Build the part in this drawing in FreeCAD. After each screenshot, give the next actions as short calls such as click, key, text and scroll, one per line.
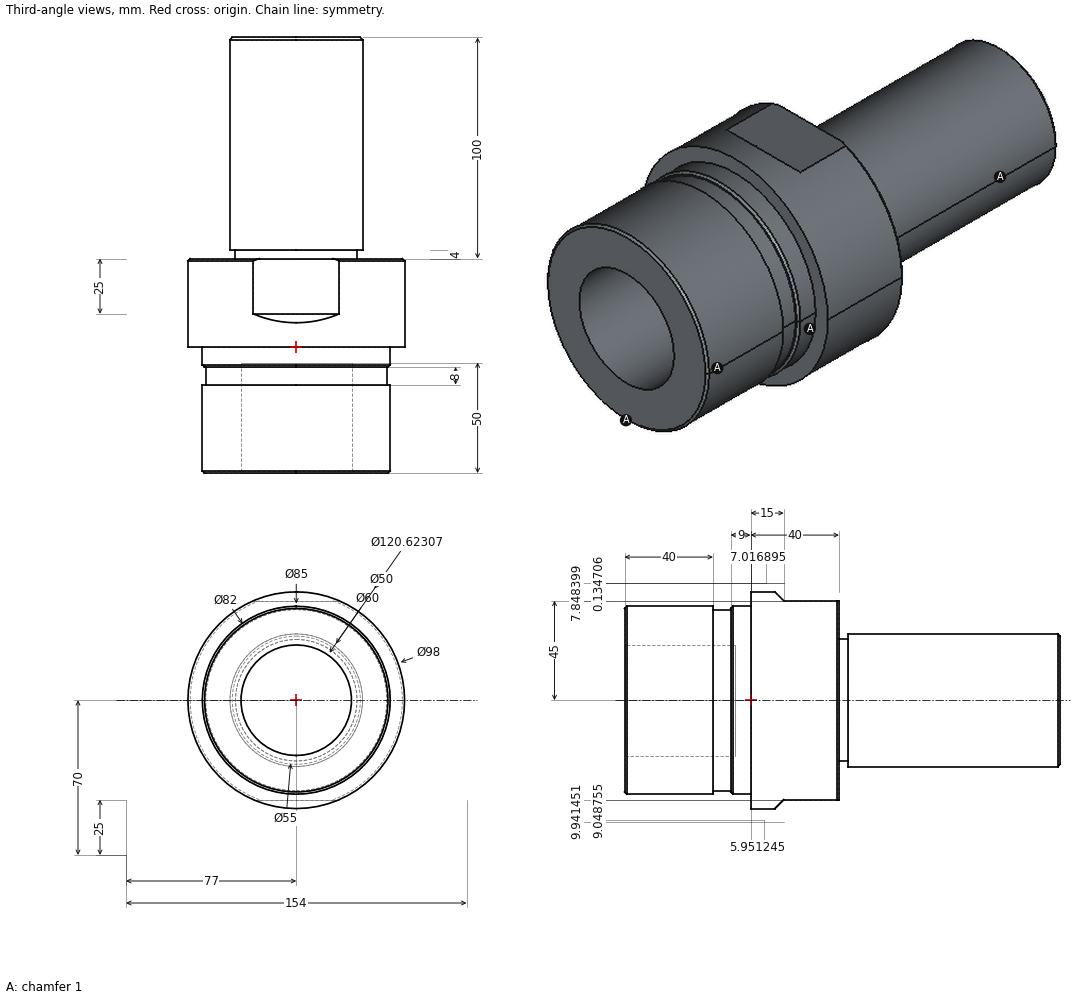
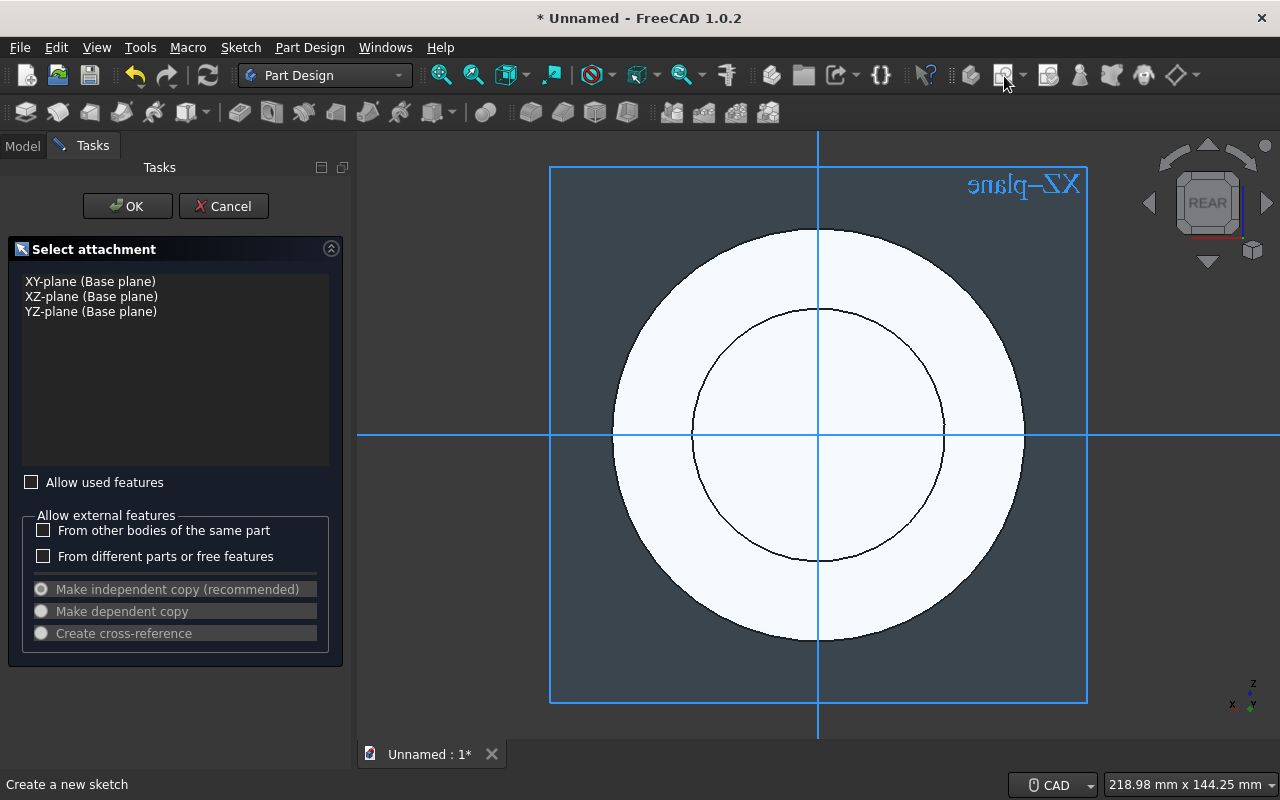
click(82, 296)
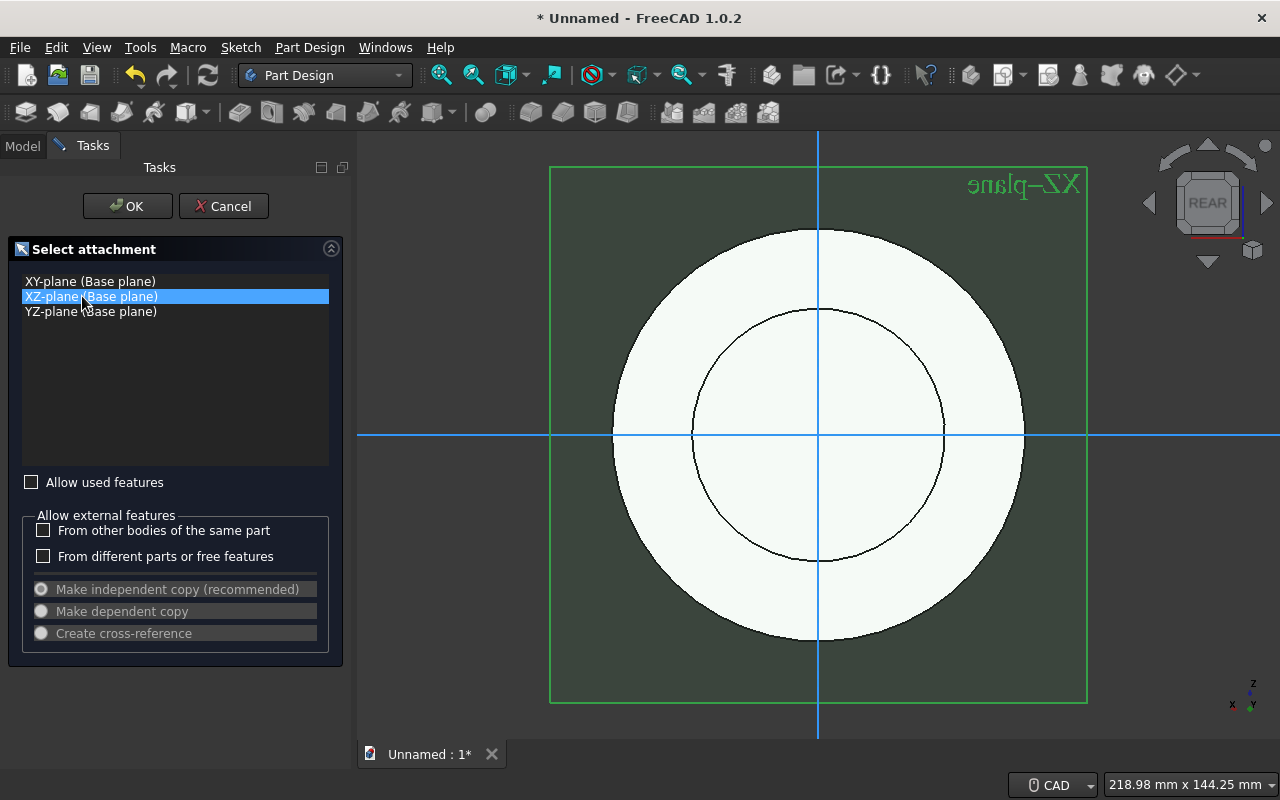
click(128, 206)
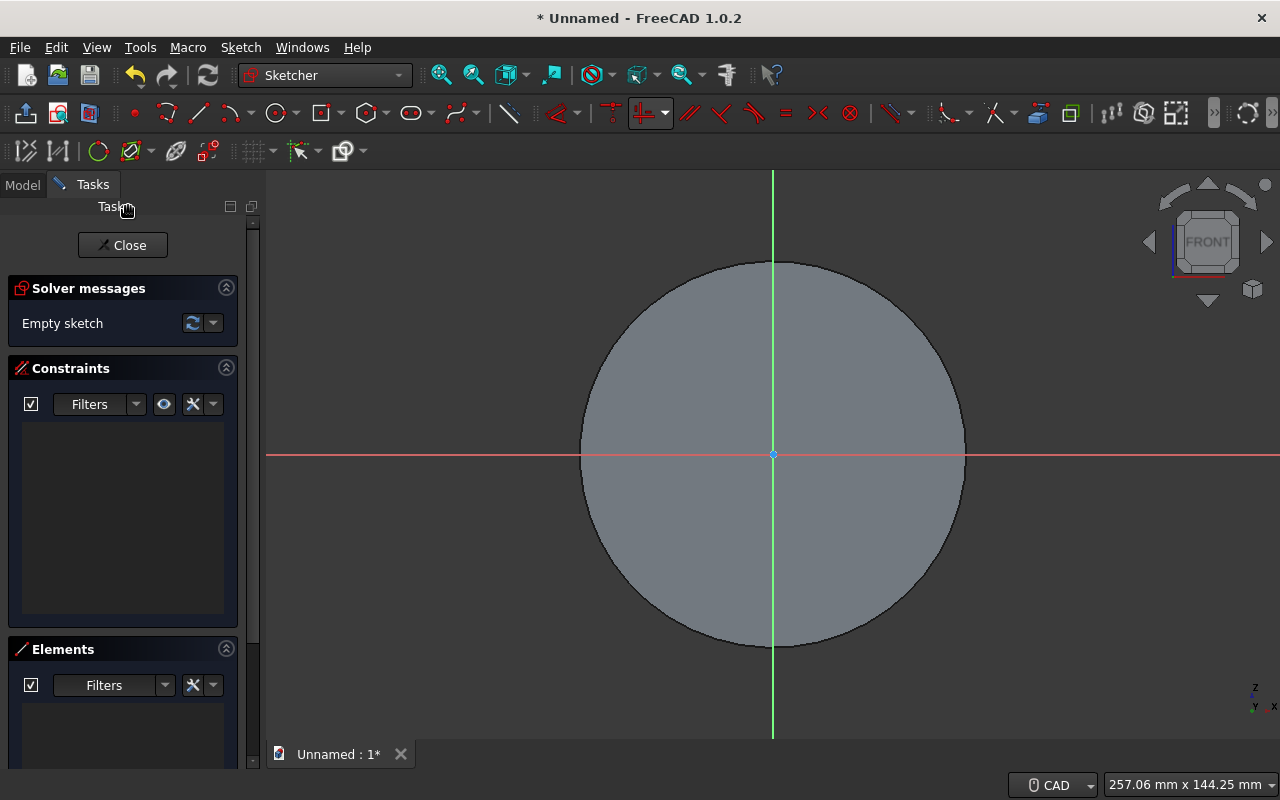
click(276, 114)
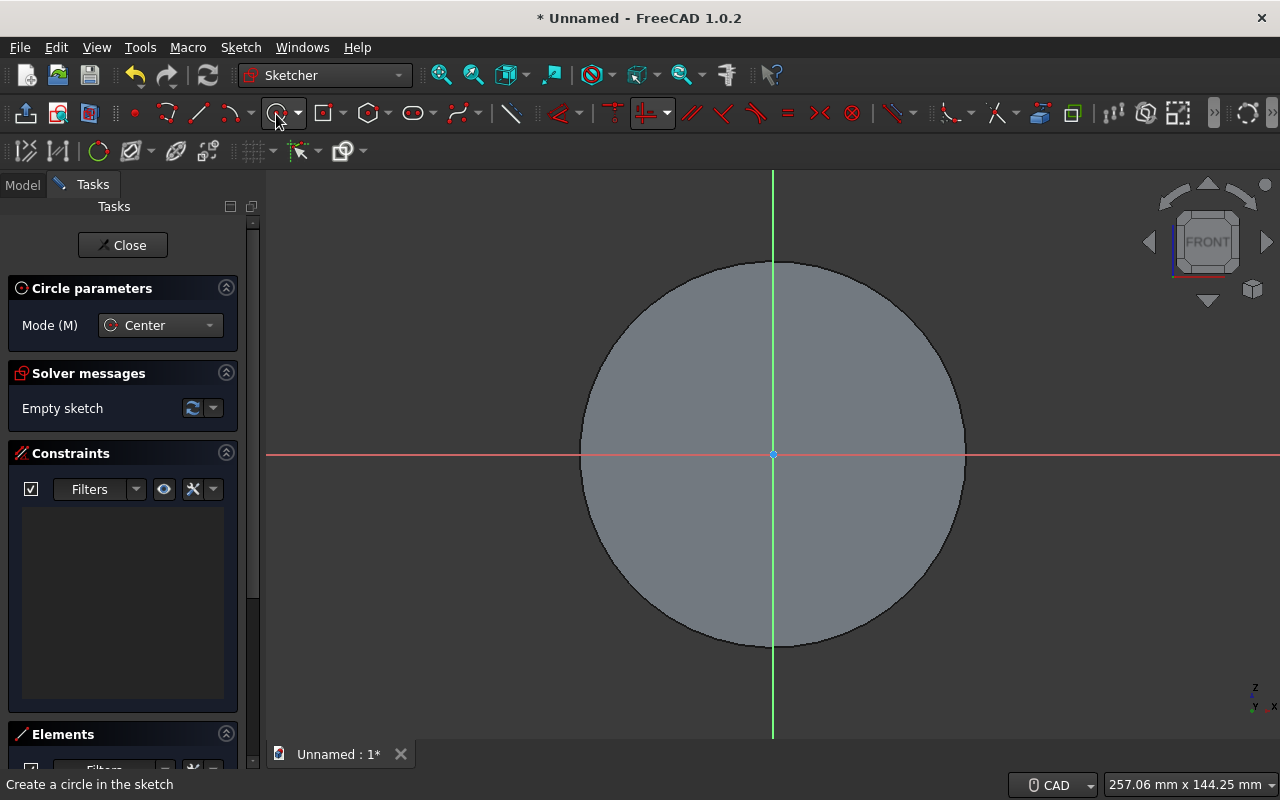
click(773, 455)
click(892, 336)
key(Escape)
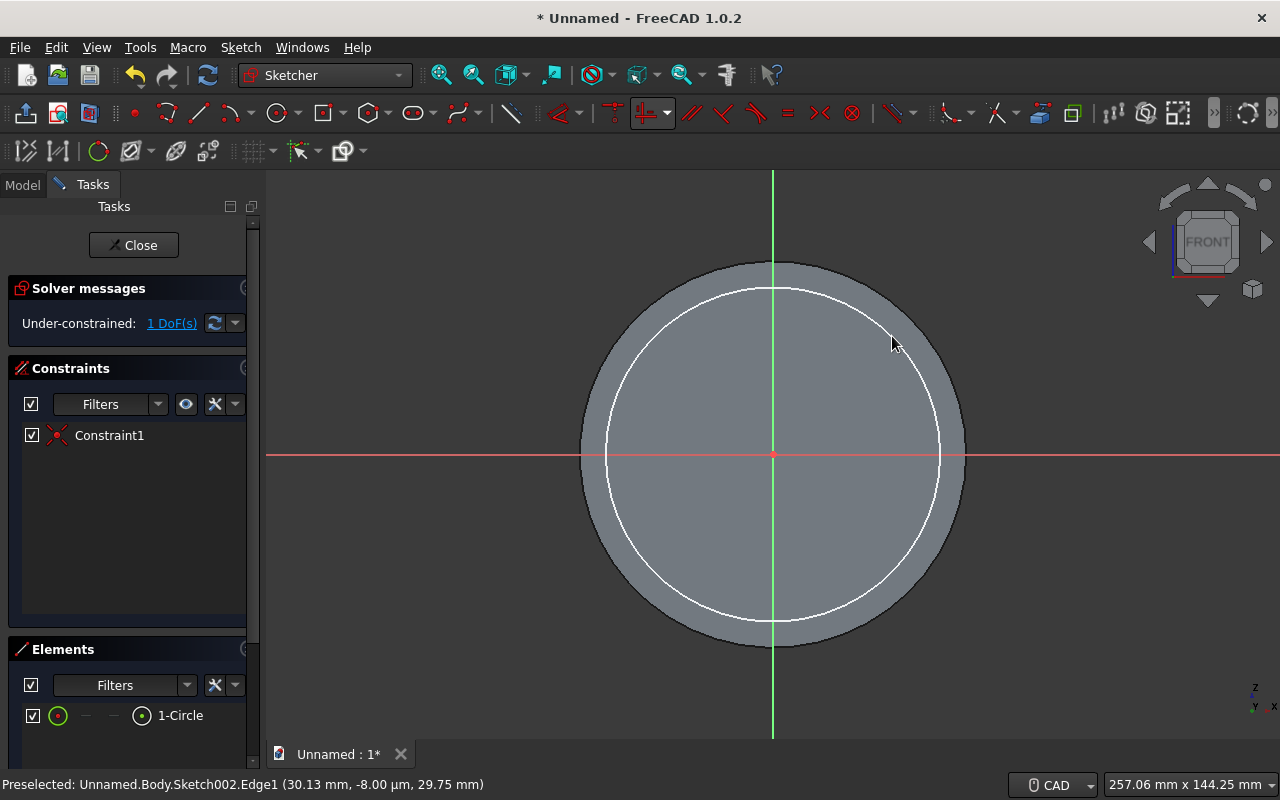
click(558, 114)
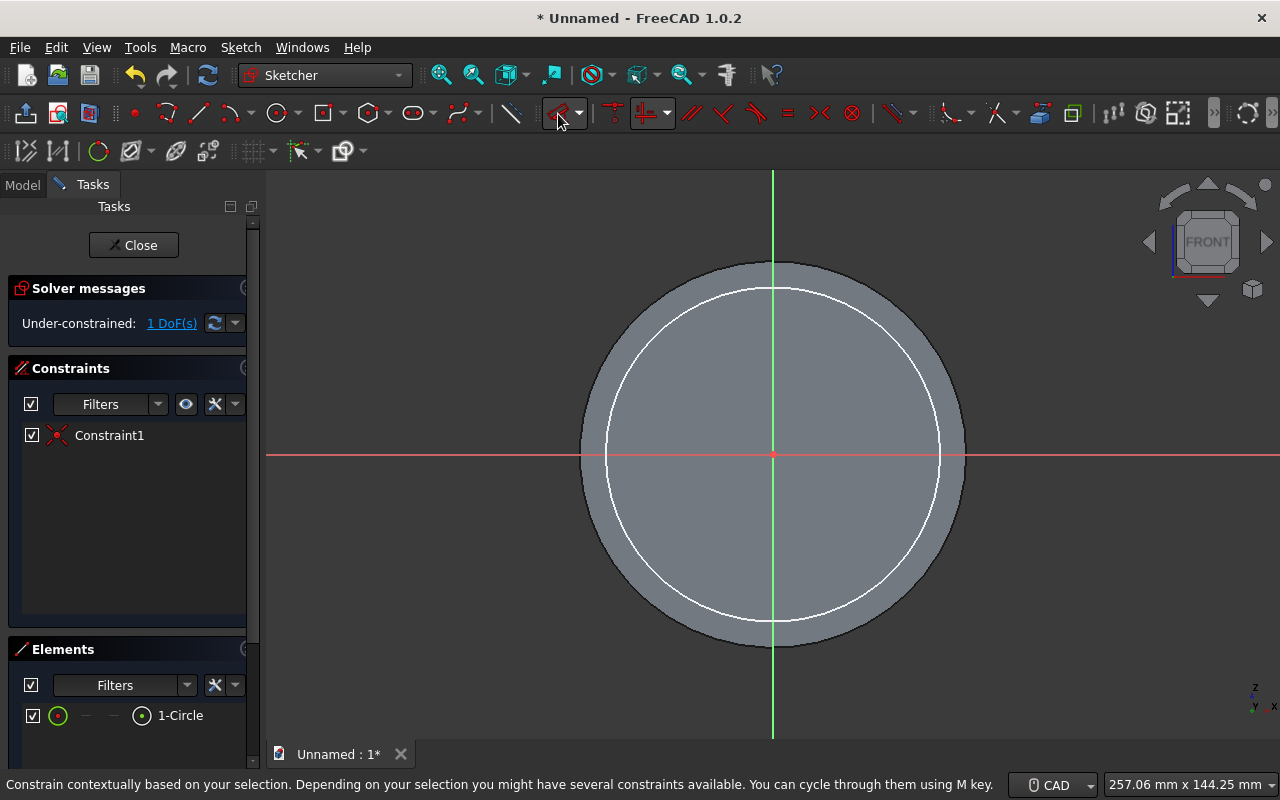
click(891, 336)
click(914, 313)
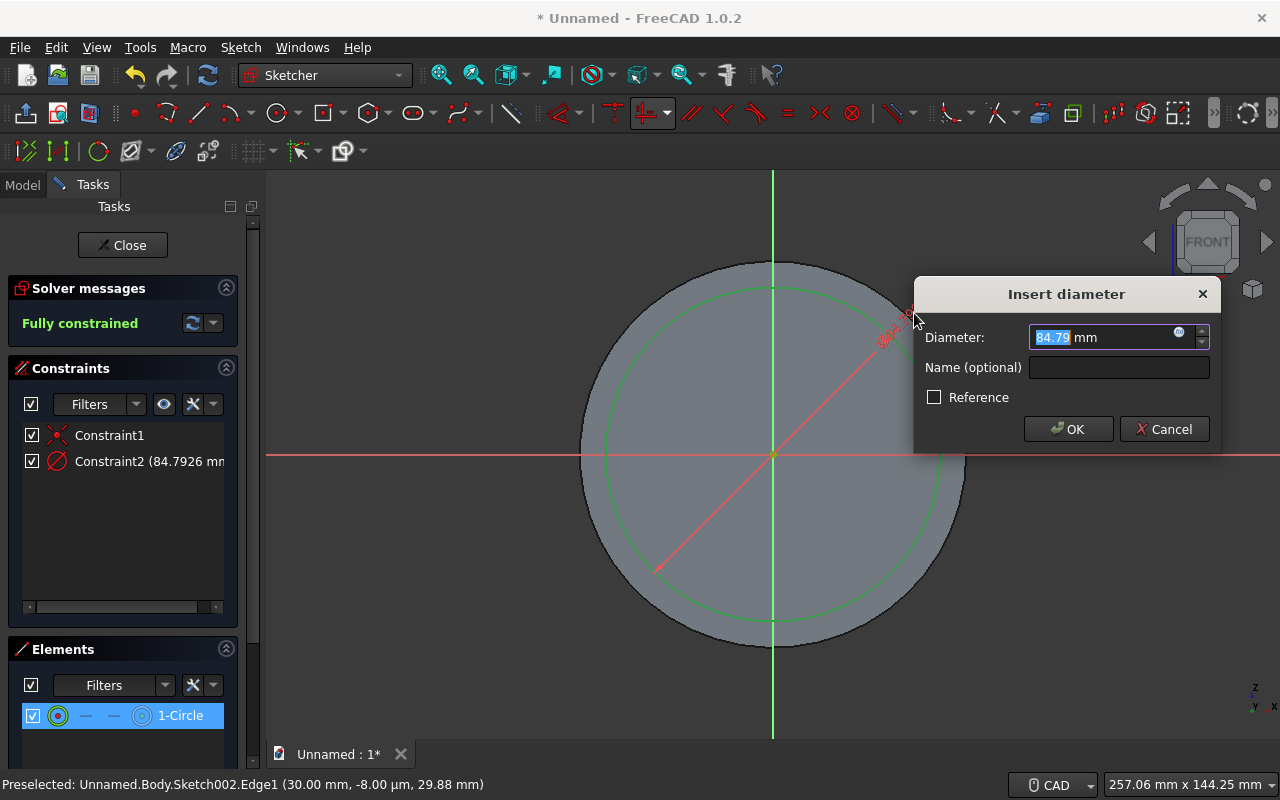
text(85)
key(Return)
key(Escape)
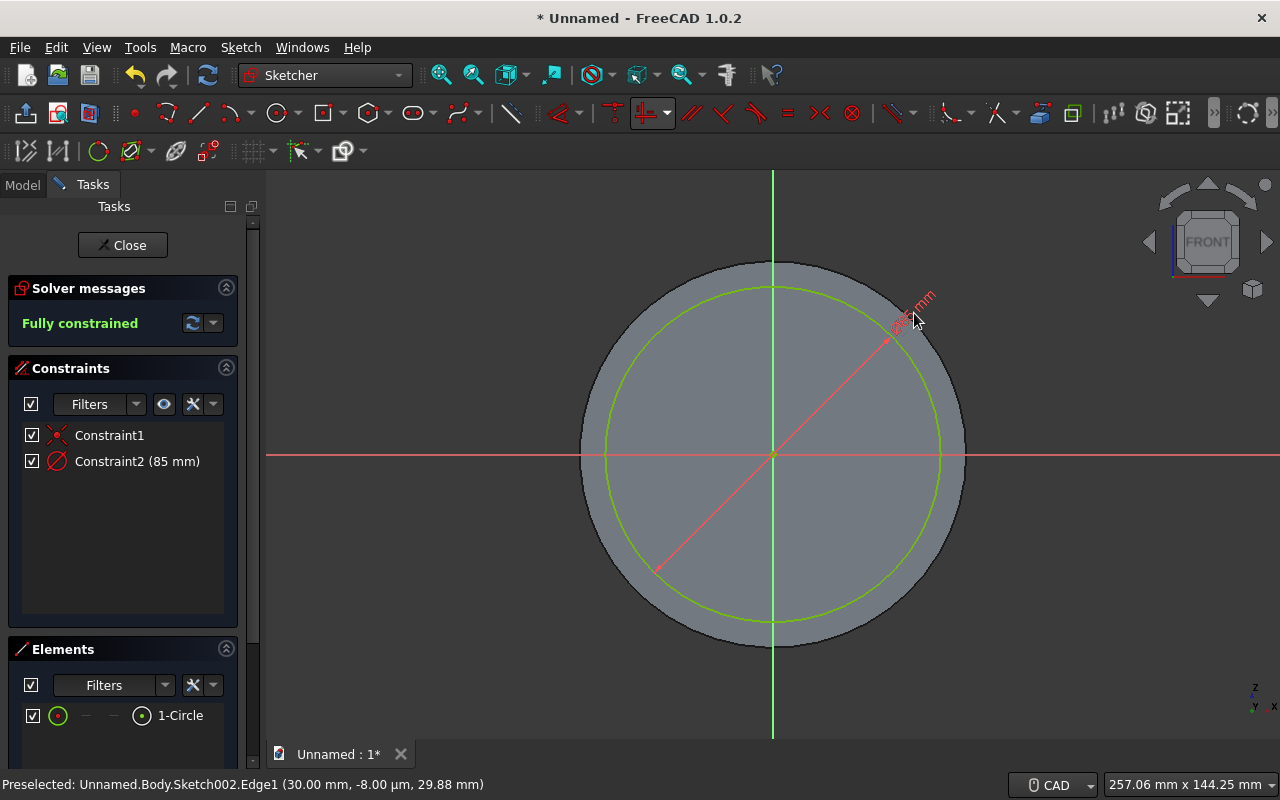
click(123, 245)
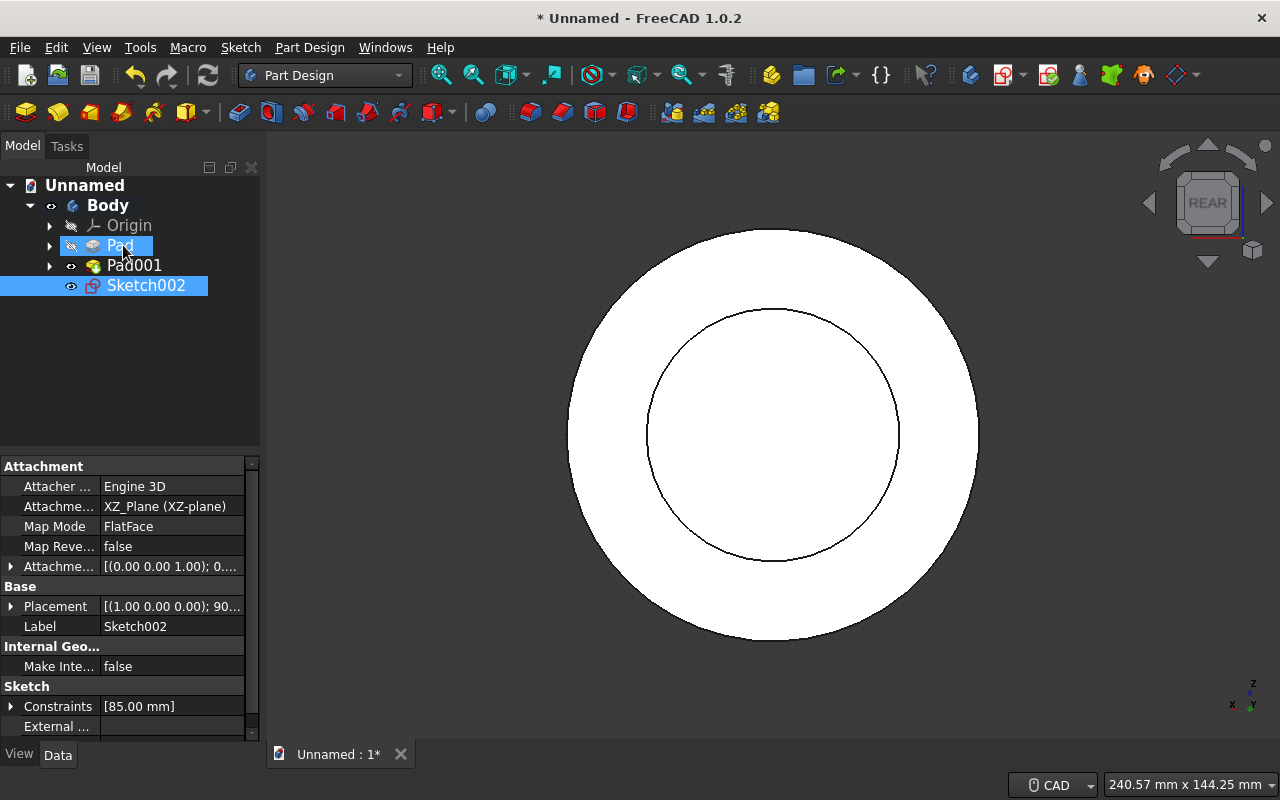
click(26, 112)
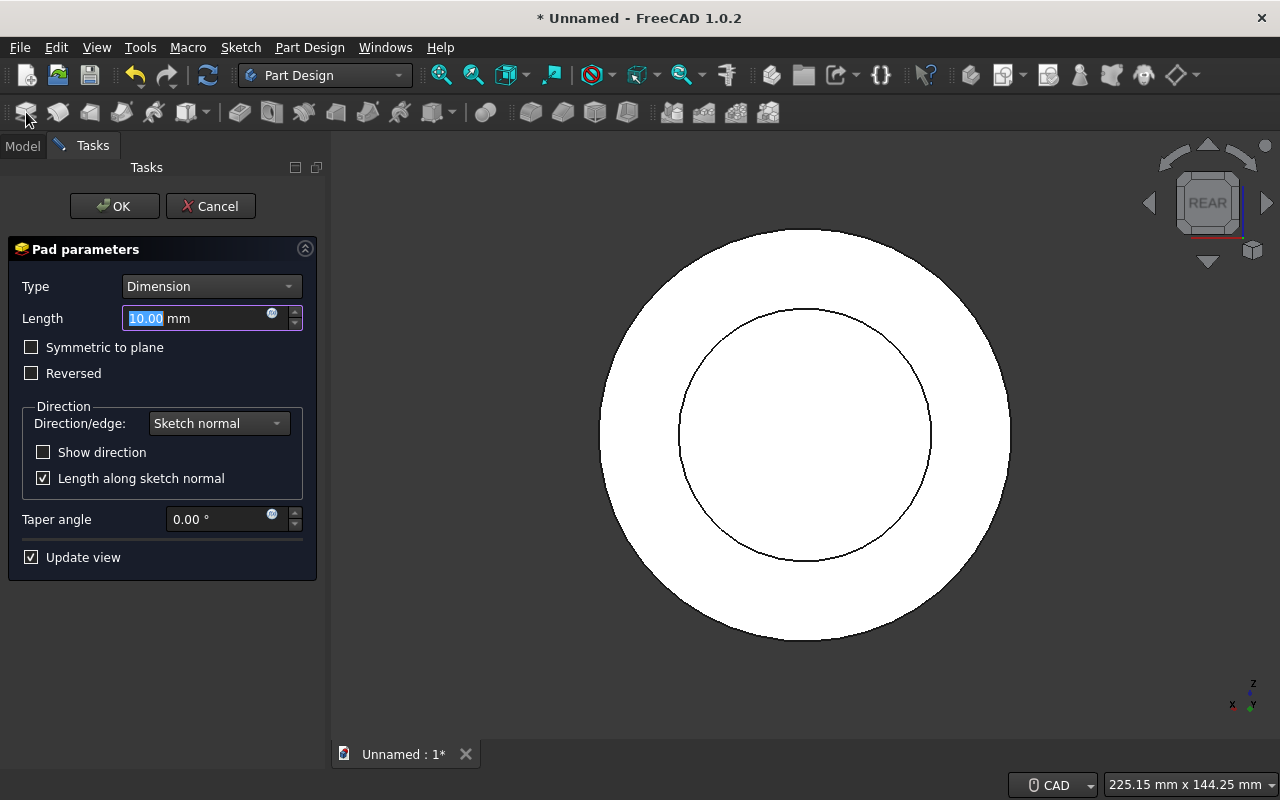
text(9)
key(Tab)